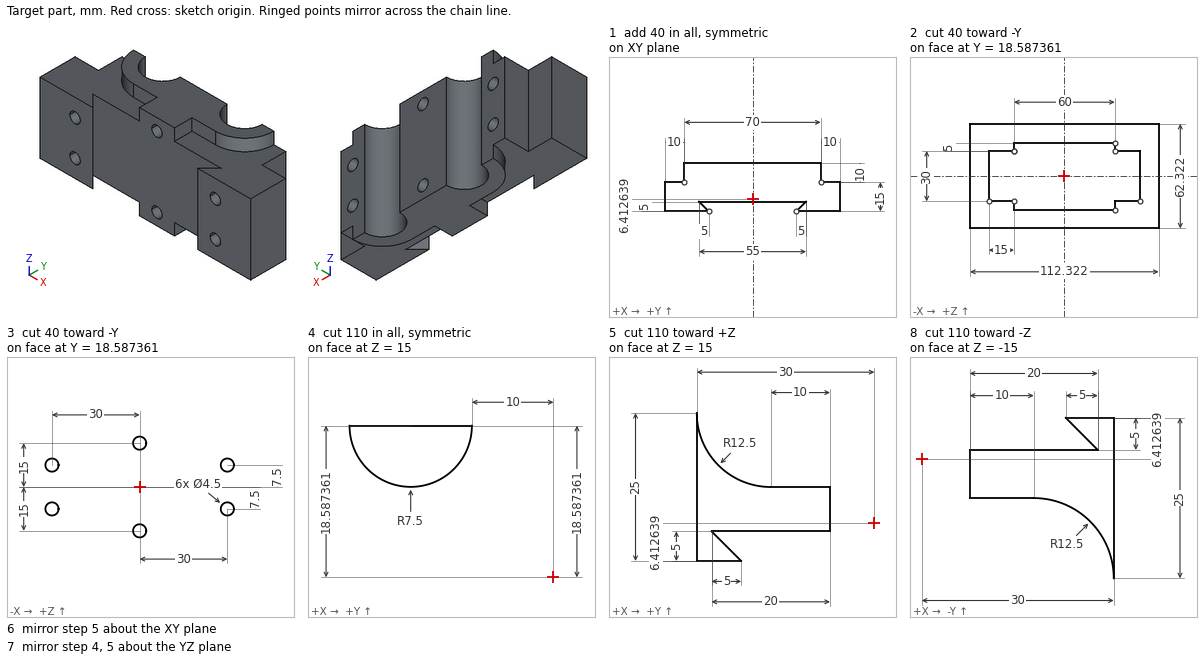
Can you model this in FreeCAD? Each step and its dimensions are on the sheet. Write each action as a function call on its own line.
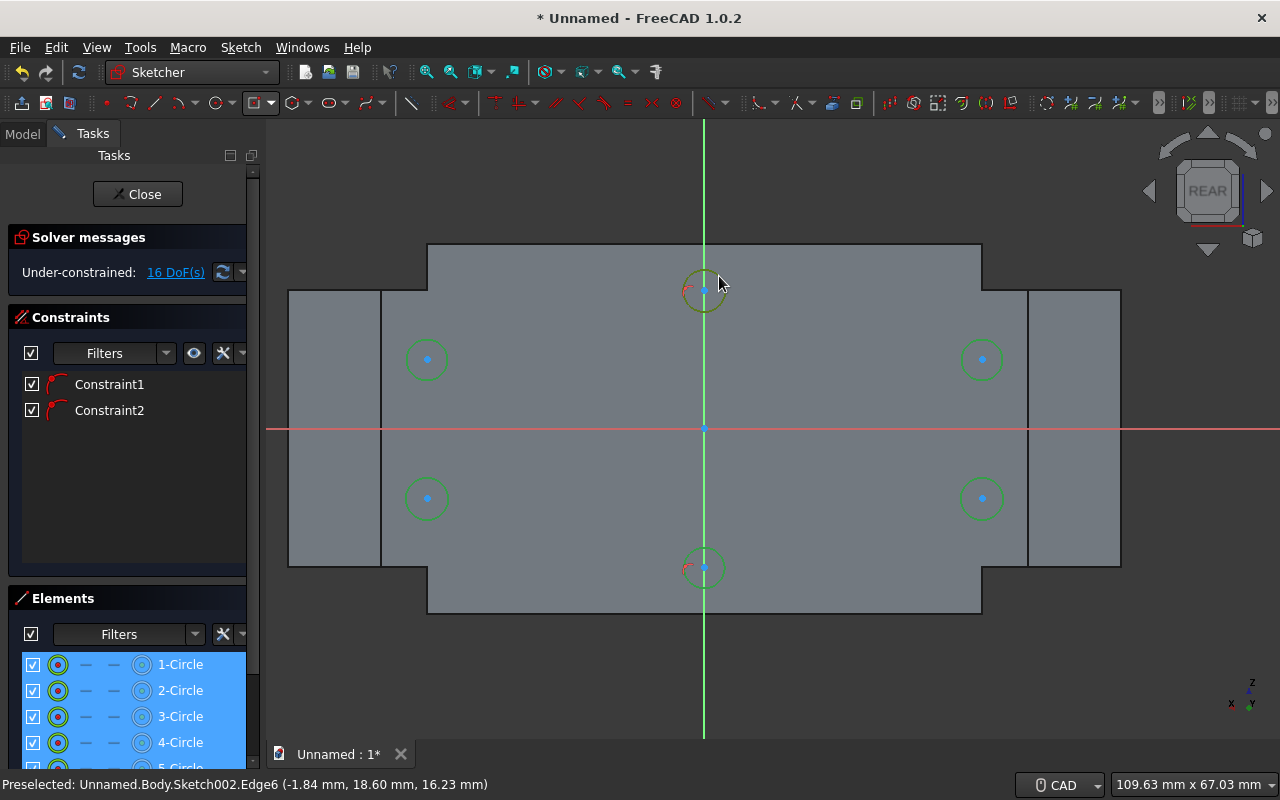
key(e)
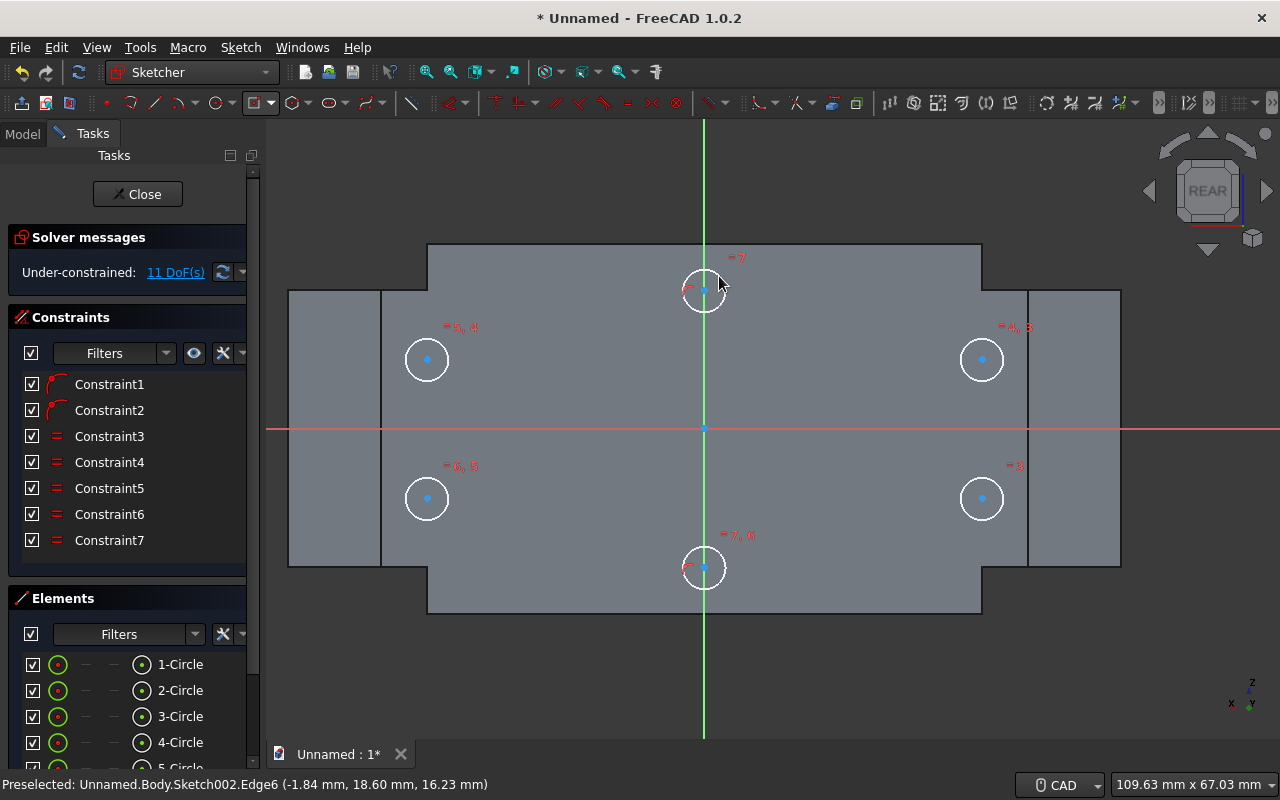
click(982, 499)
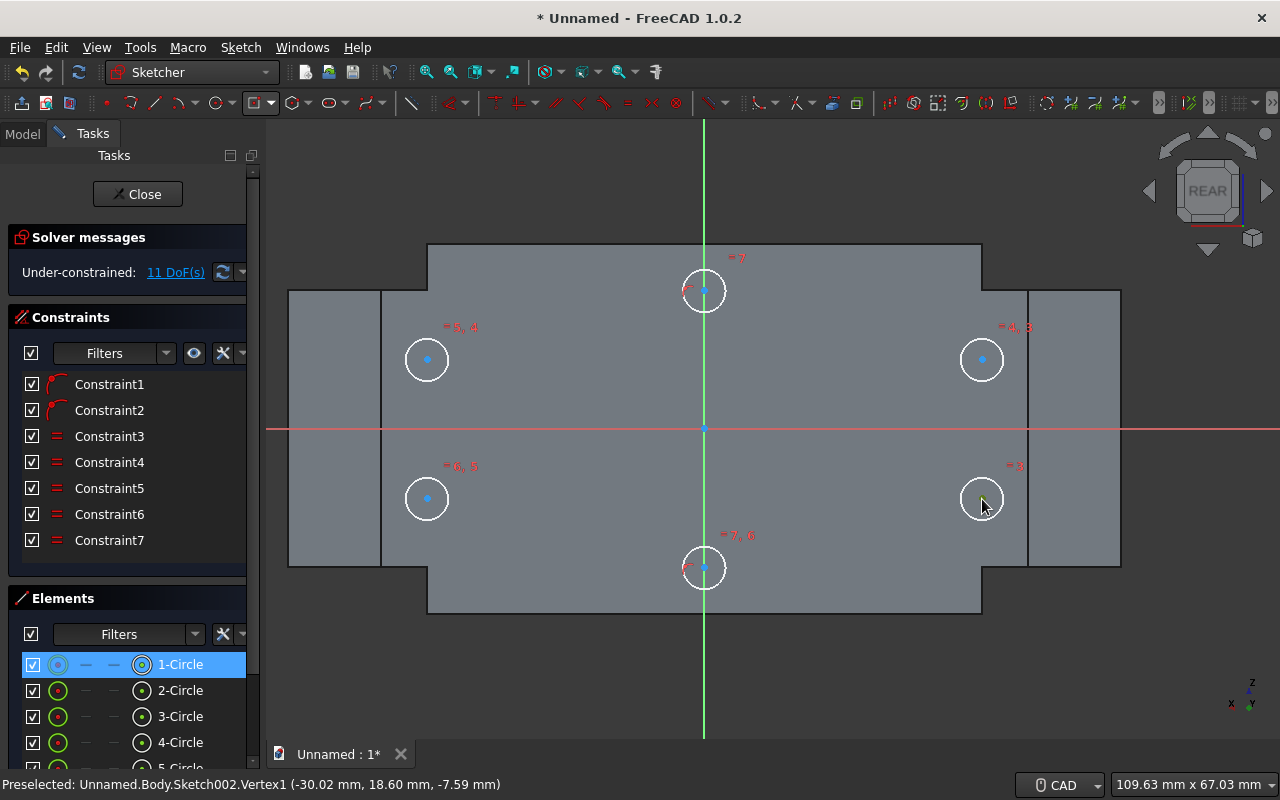
click(982, 360)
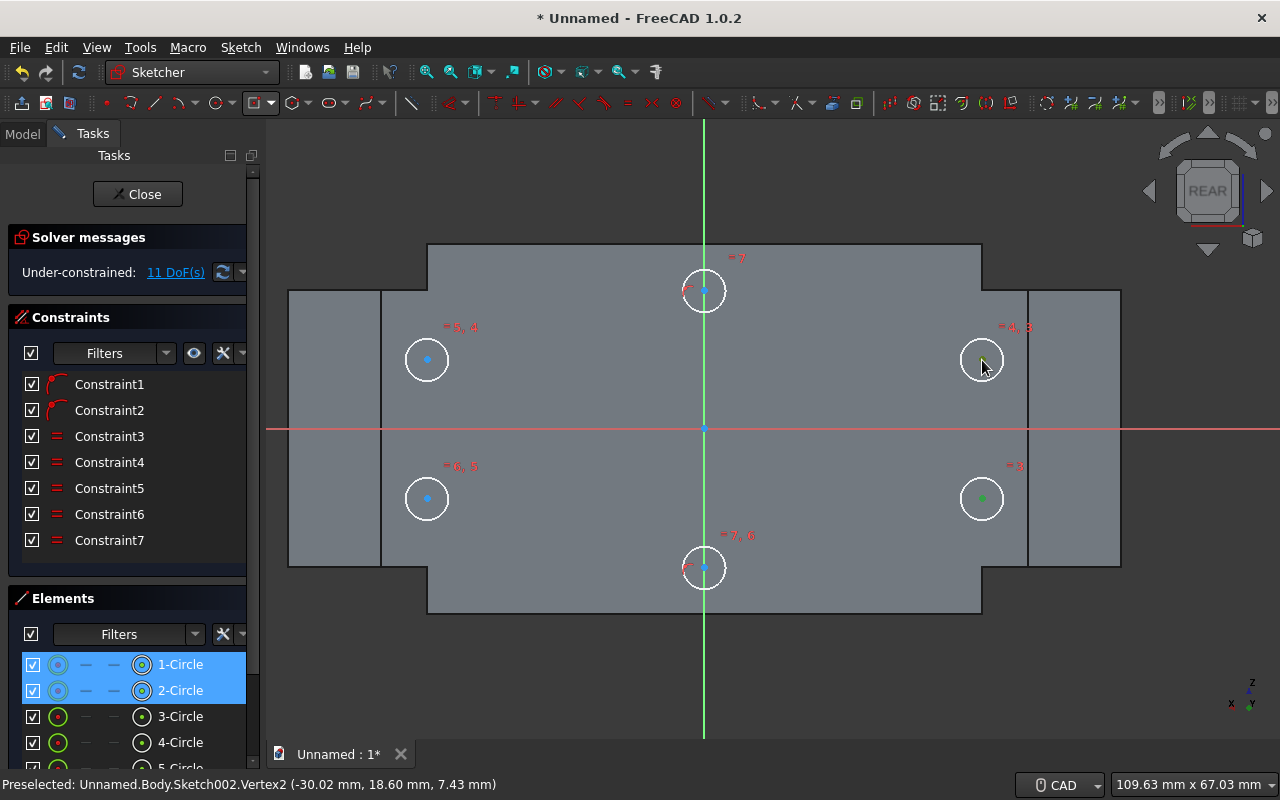
key(v)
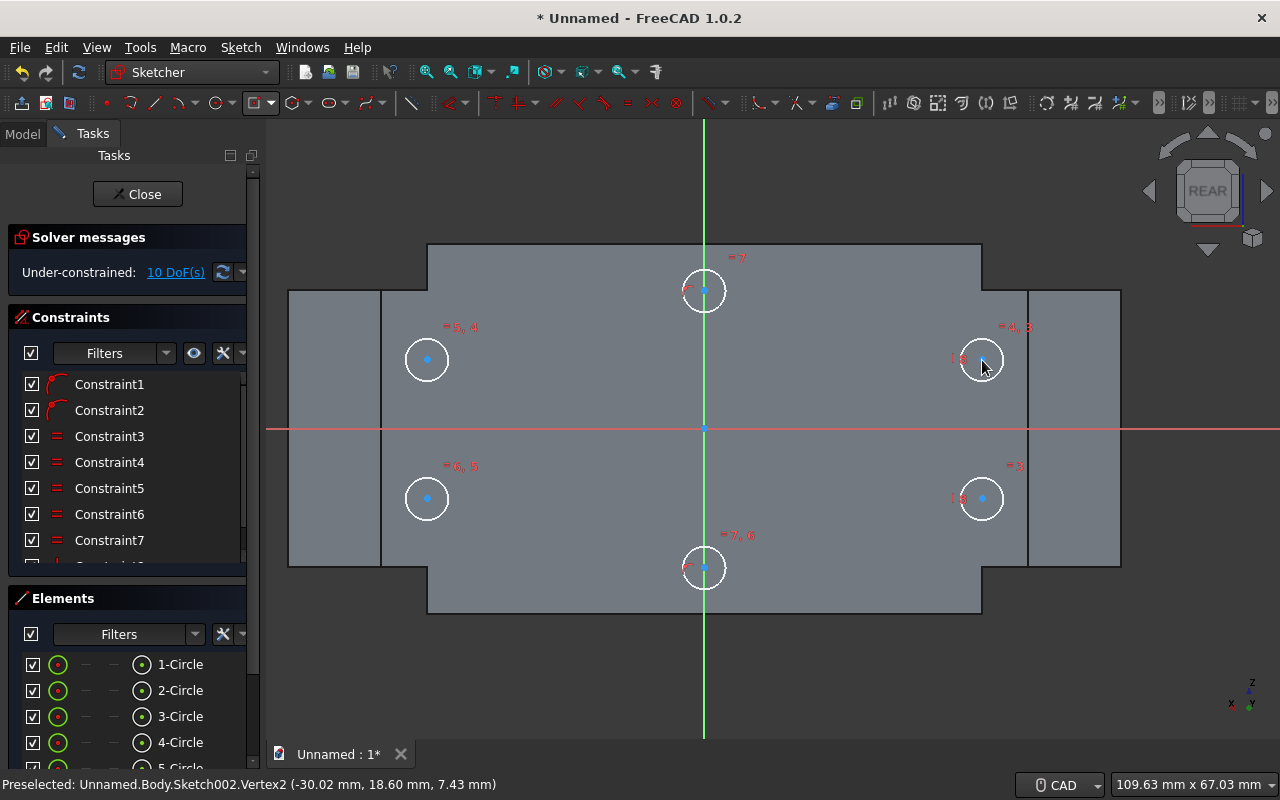
click(982, 360)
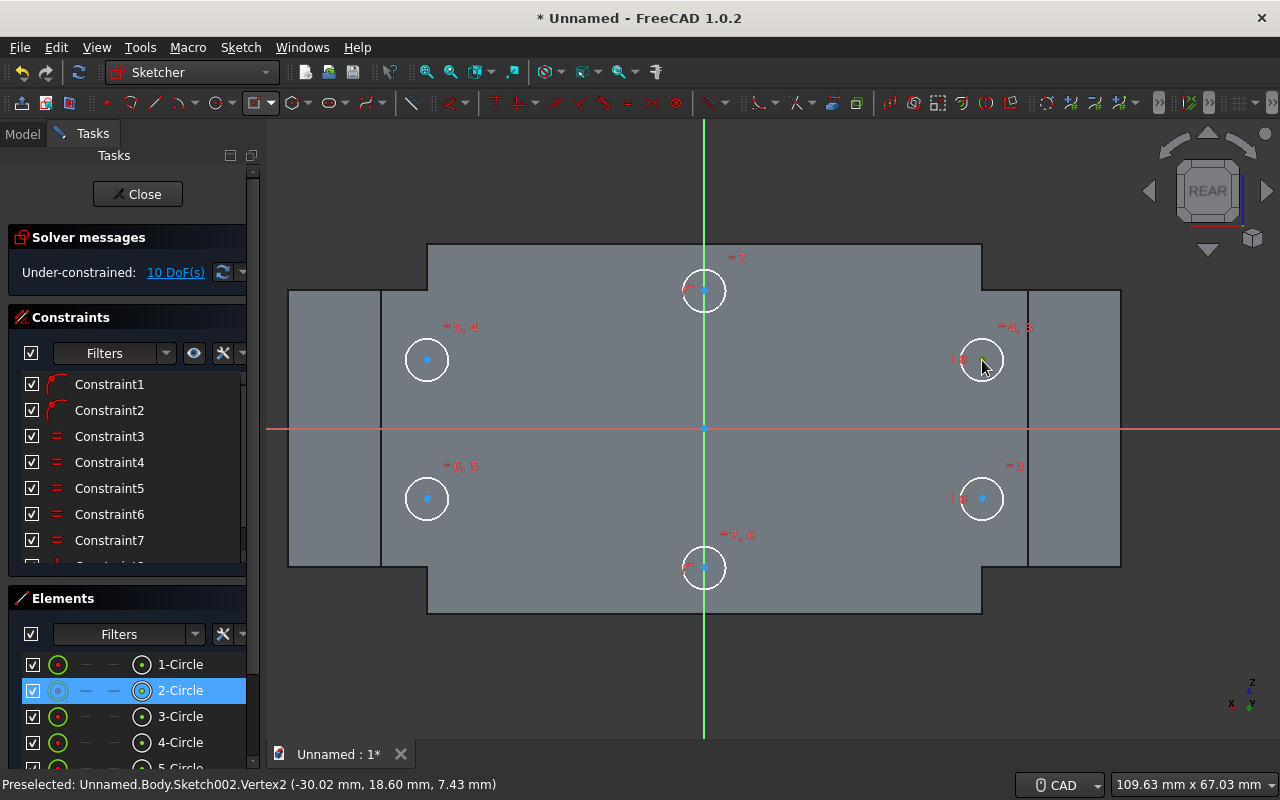
click(427, 360)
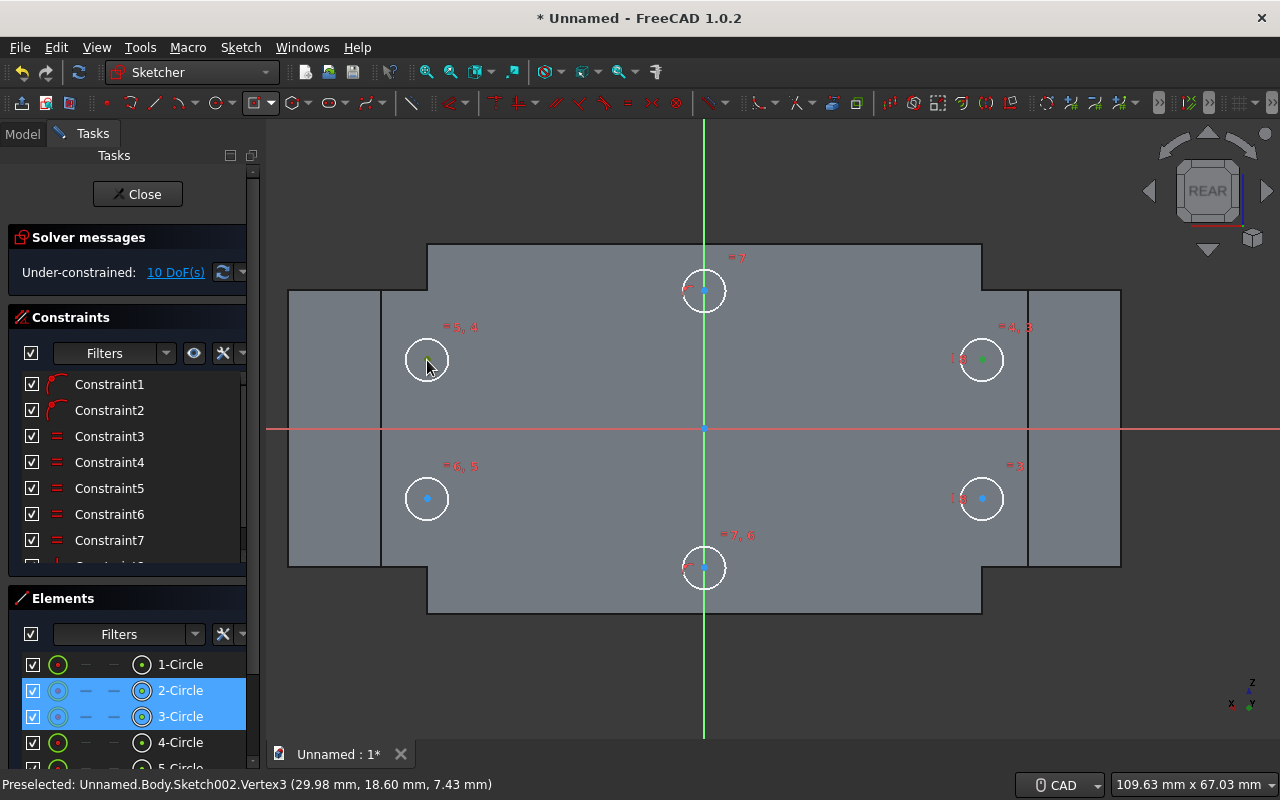
key(h)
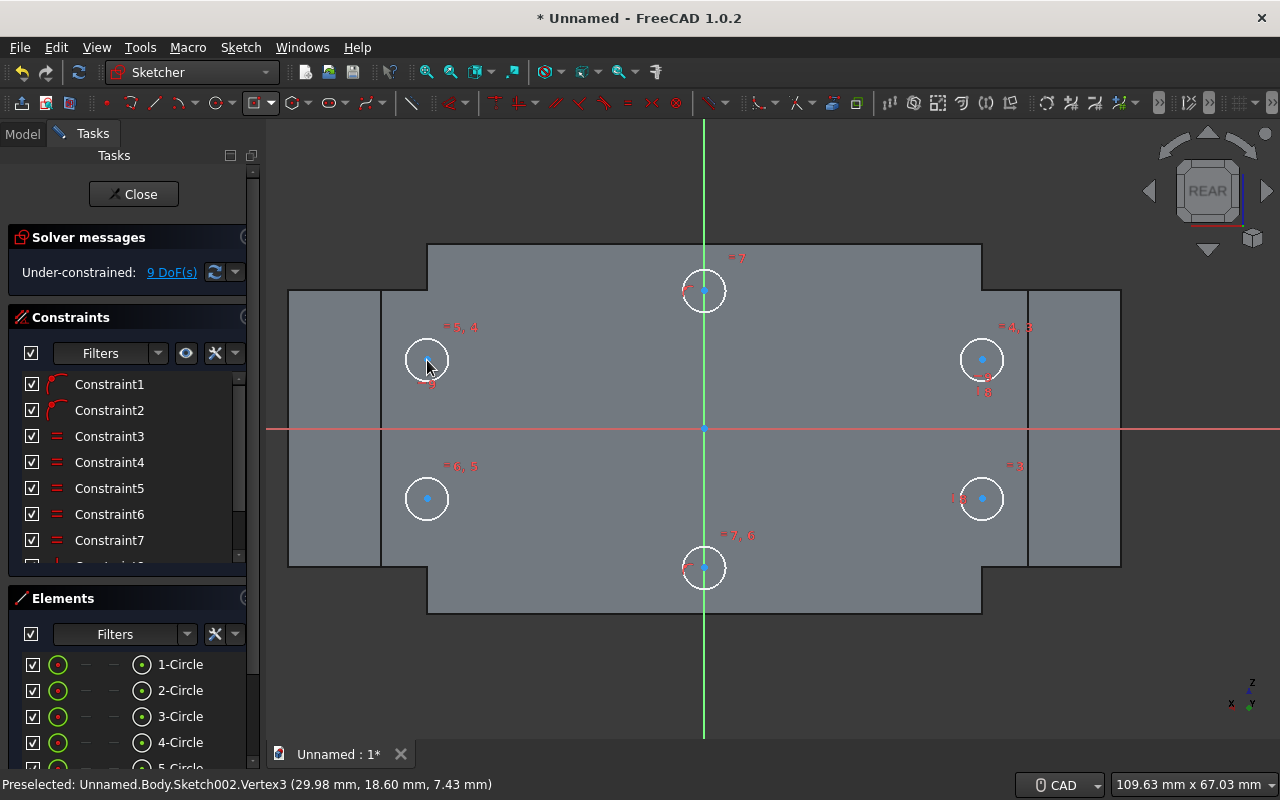
click(427, 360)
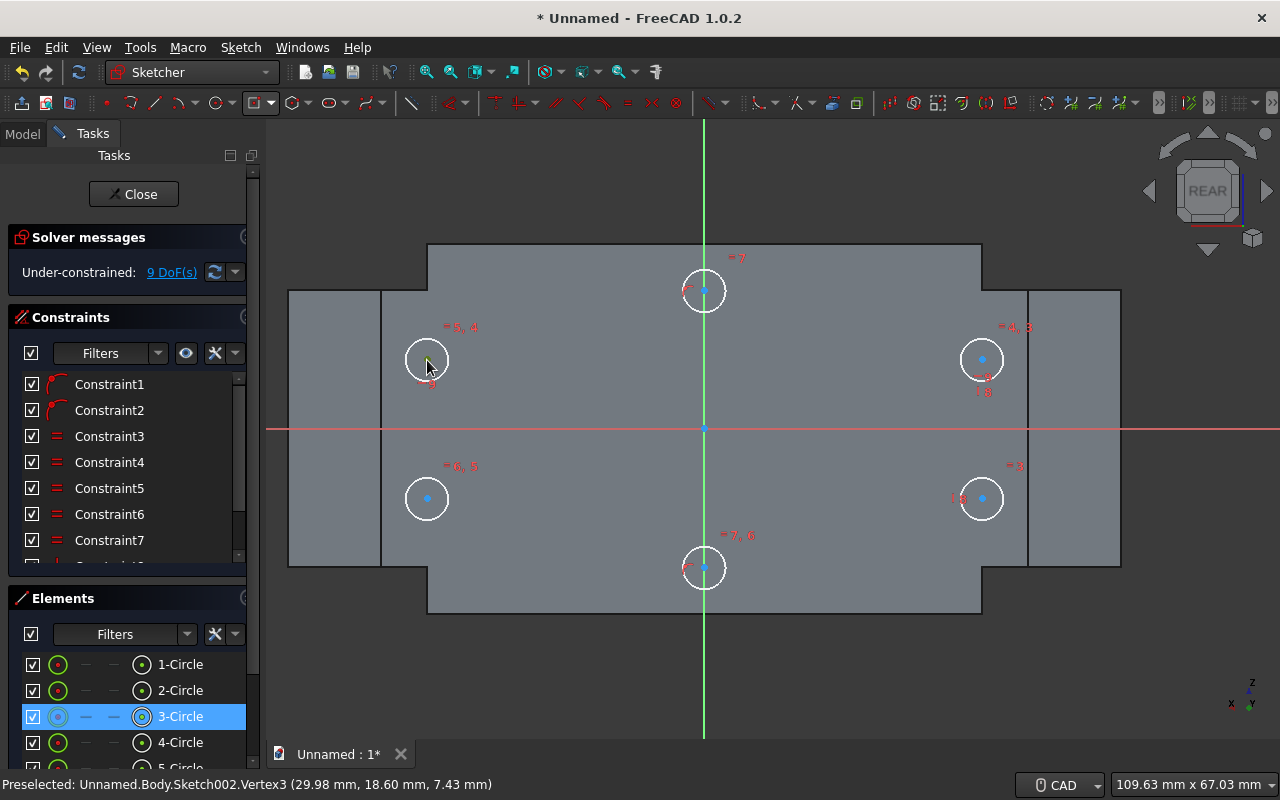
click(427, 499)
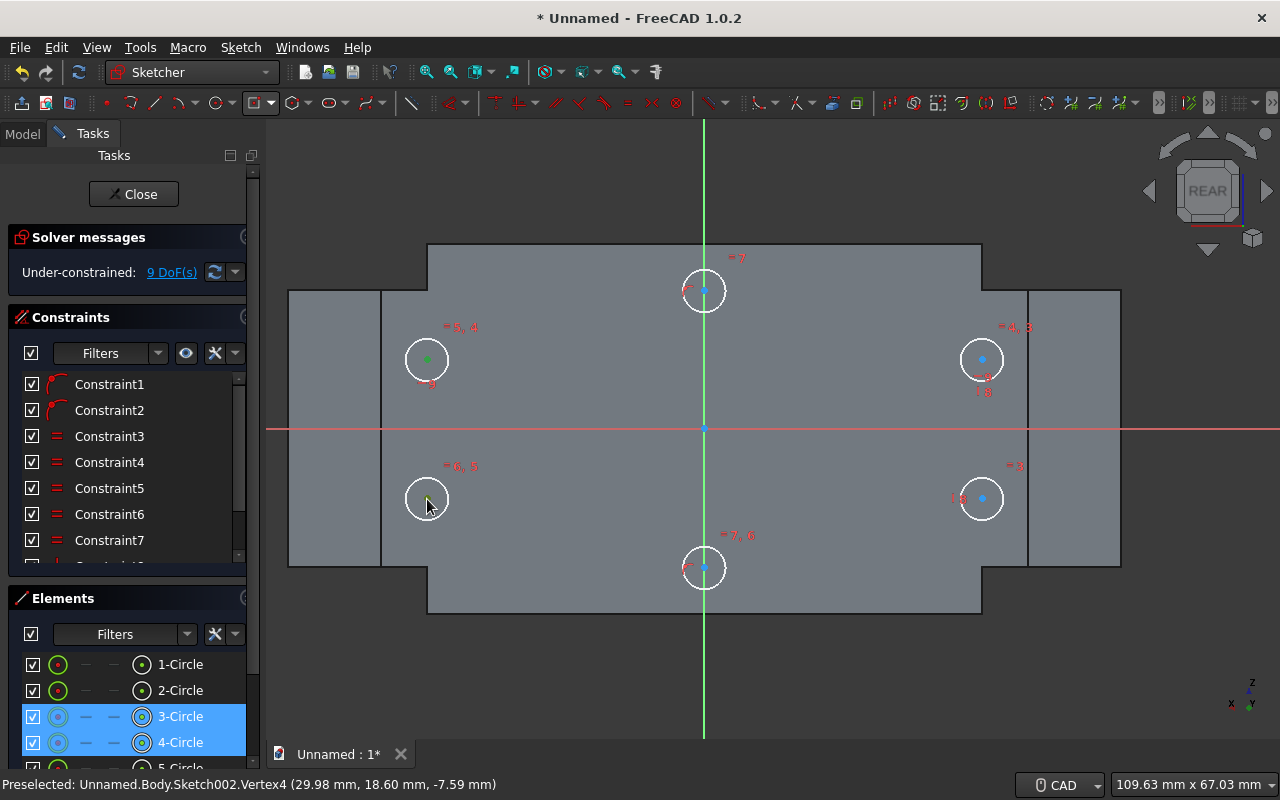
key(v)